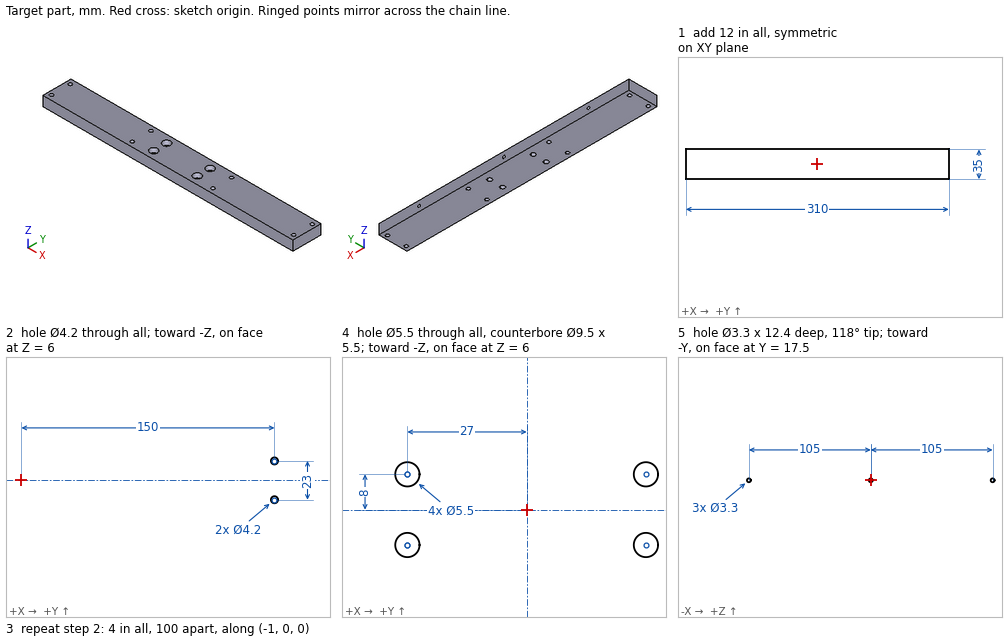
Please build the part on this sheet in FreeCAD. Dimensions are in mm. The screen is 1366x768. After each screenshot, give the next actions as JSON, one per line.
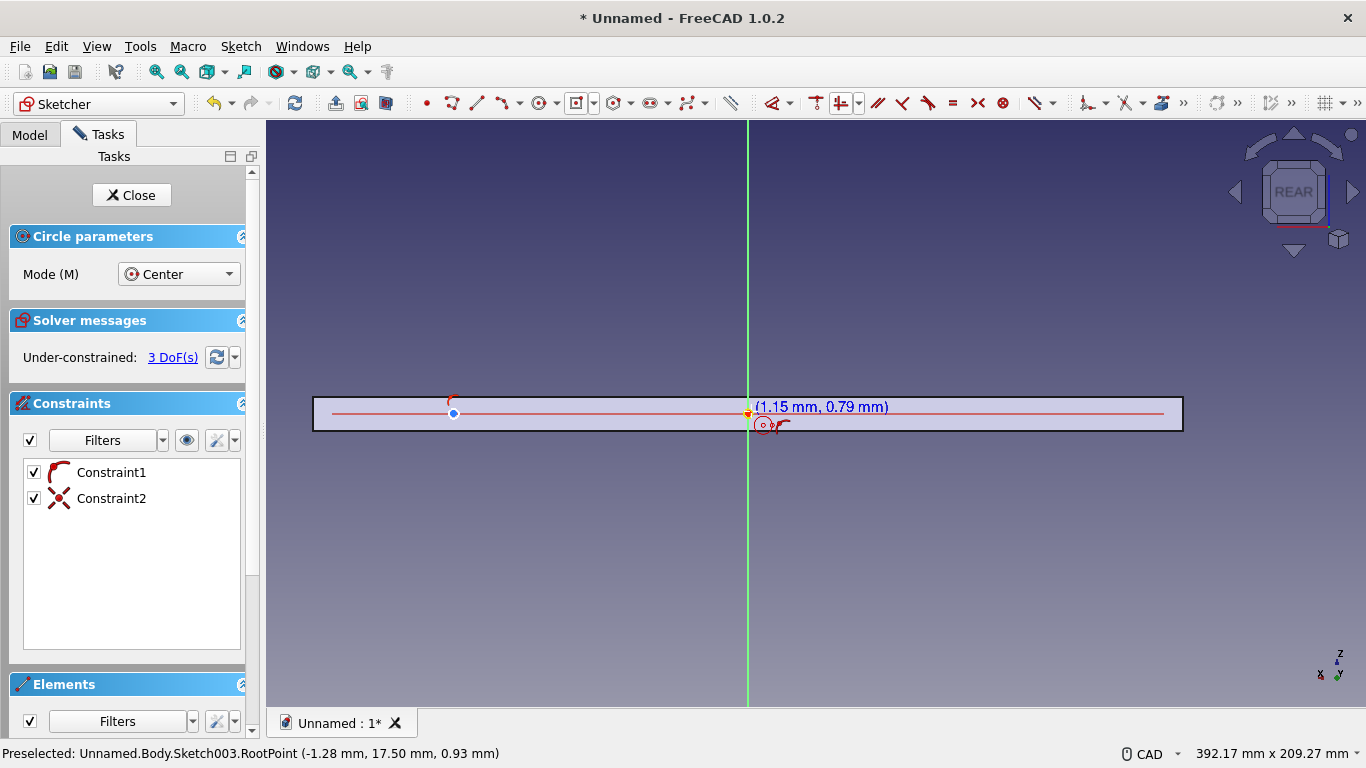
{"action": "scroll", "coordinate": [1043, 414], "scroll_direction": "up", "scroll_amount": 8}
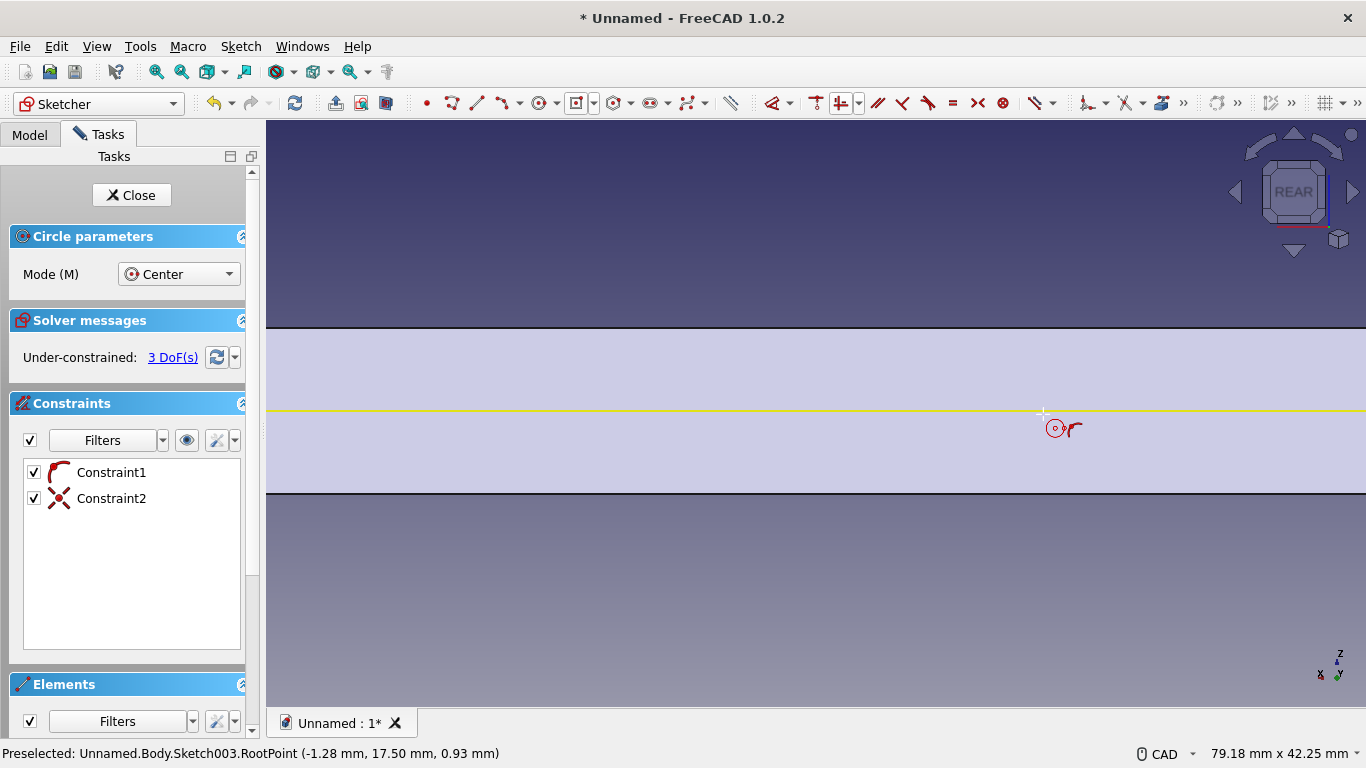
{"action": "scroll", "coordinate": [1043, 414], "scroll_direction": "down", "scroll_amount": 8}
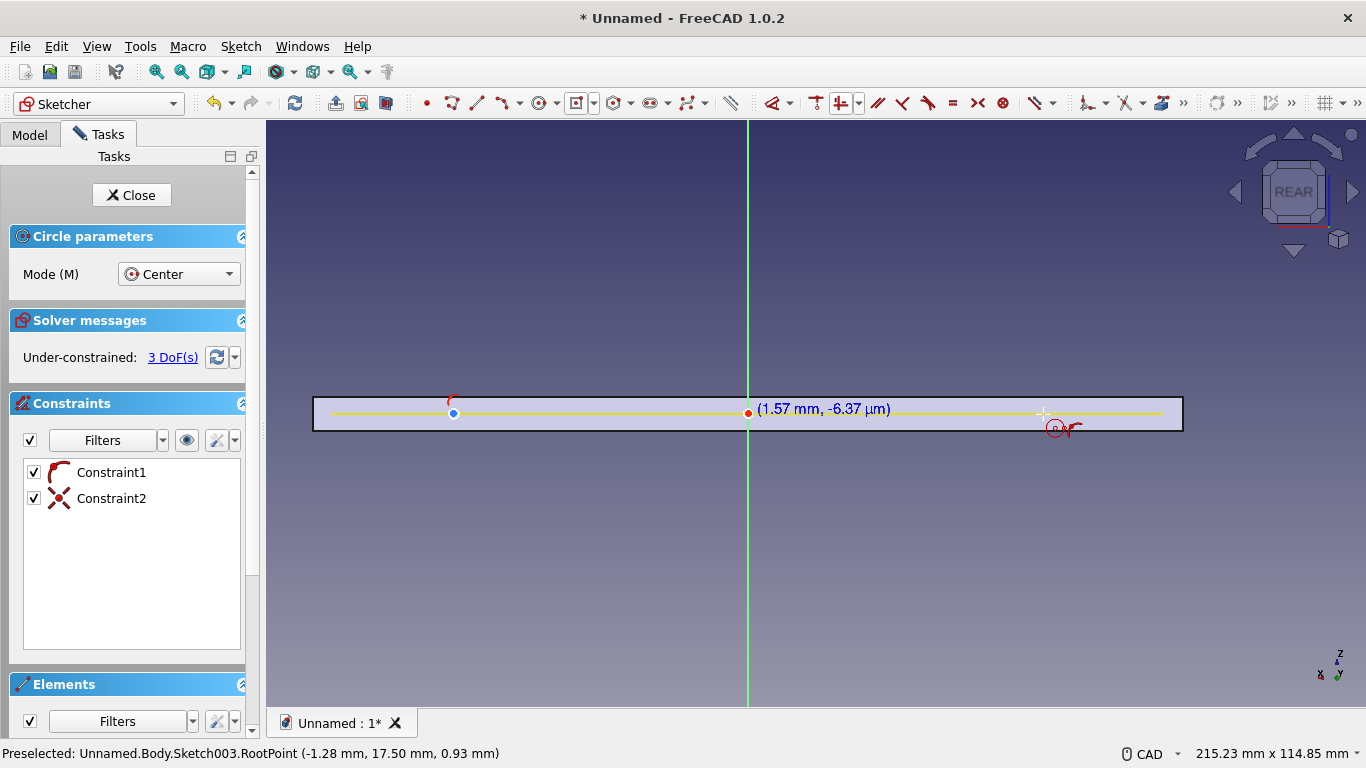
{"action": "left_click", "coordinate": [1043, 414]}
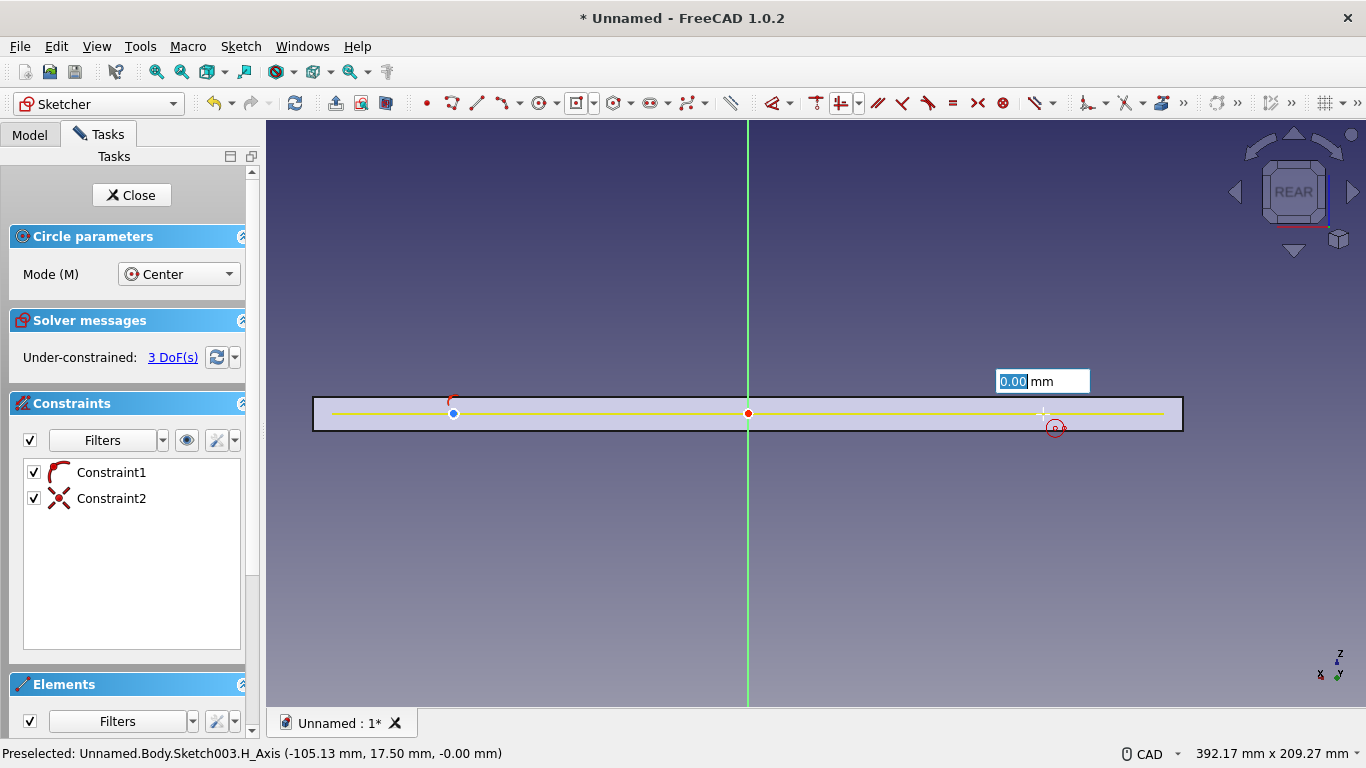
{"action": "scroll", "coordinate": [1041, 418], "scroll_direction": "up", "scroll_amount": 7}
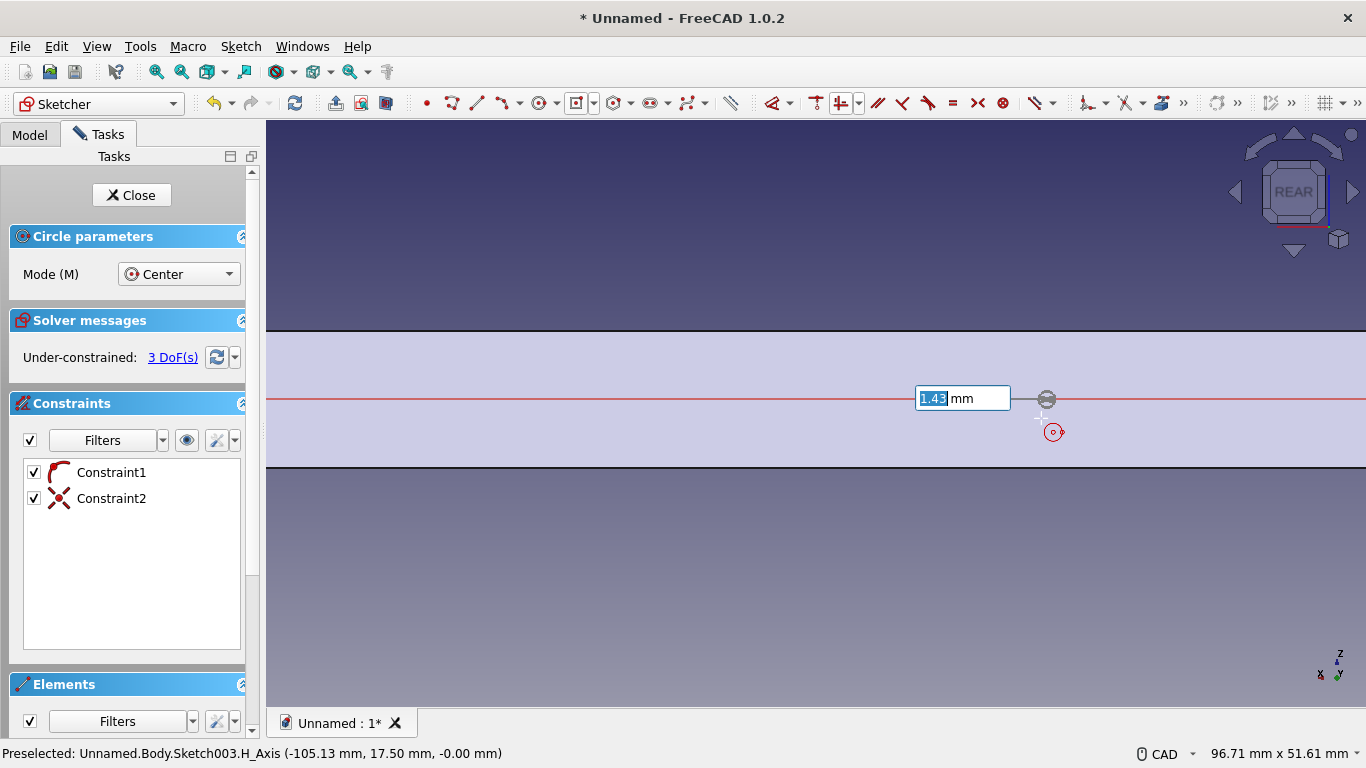
{"action": "left_click", "coordinate": [1039, 417]}
{"action": "key", "text": "Escape"}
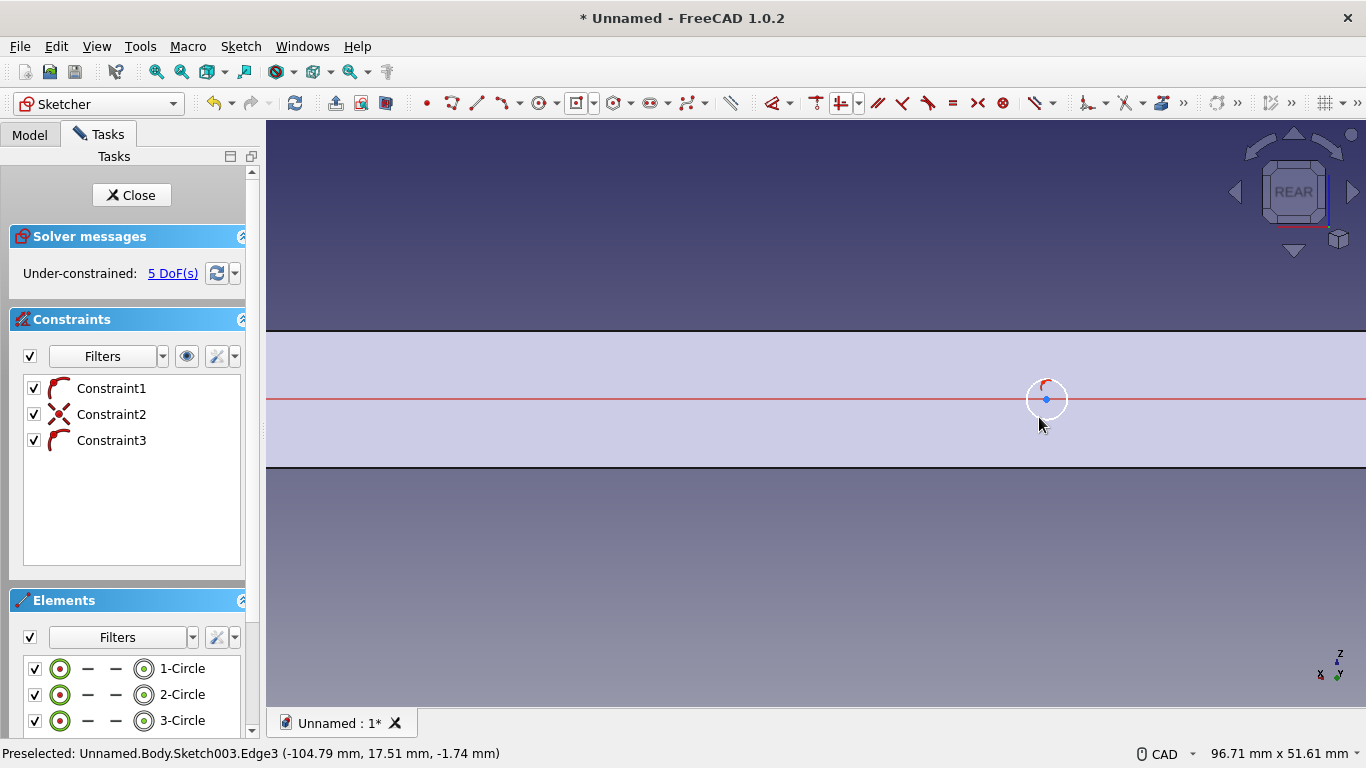
{"action": "scroll", "coordinate": [1041, 418], "scroll_direction": "down", "scroll_amount": 7}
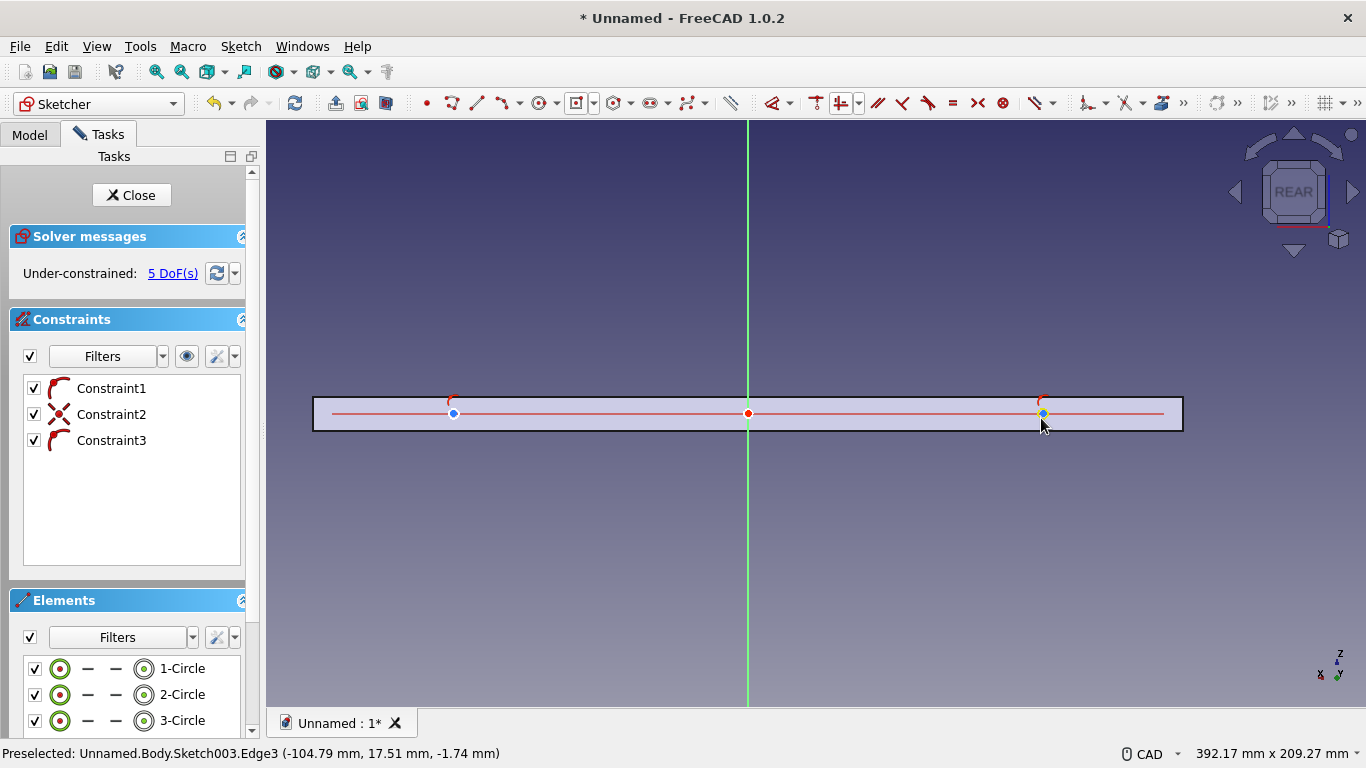
{"action": "scroll", "coordinate": [457, 410], "scroll_direction": "up", "scroll_amount": 7}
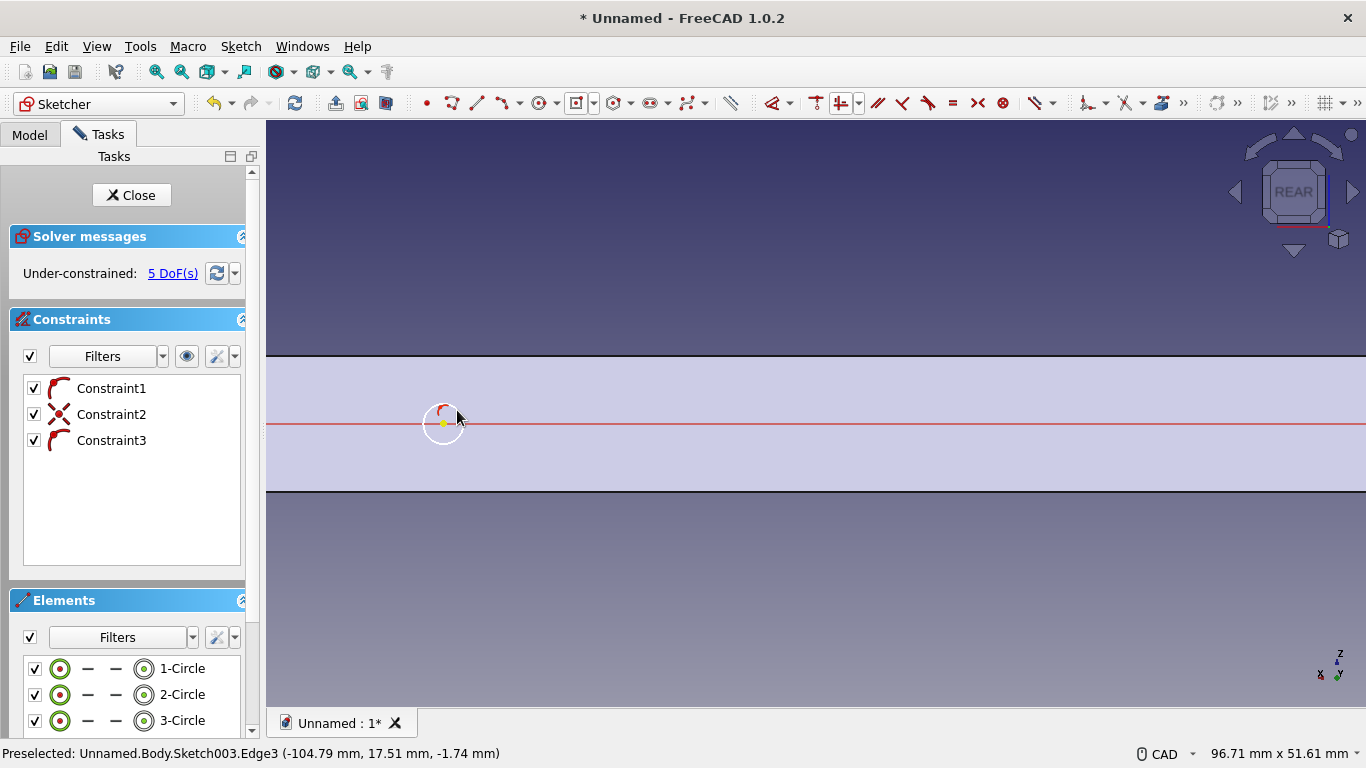
{"action": "left_click", "coordinate": [458, 410]}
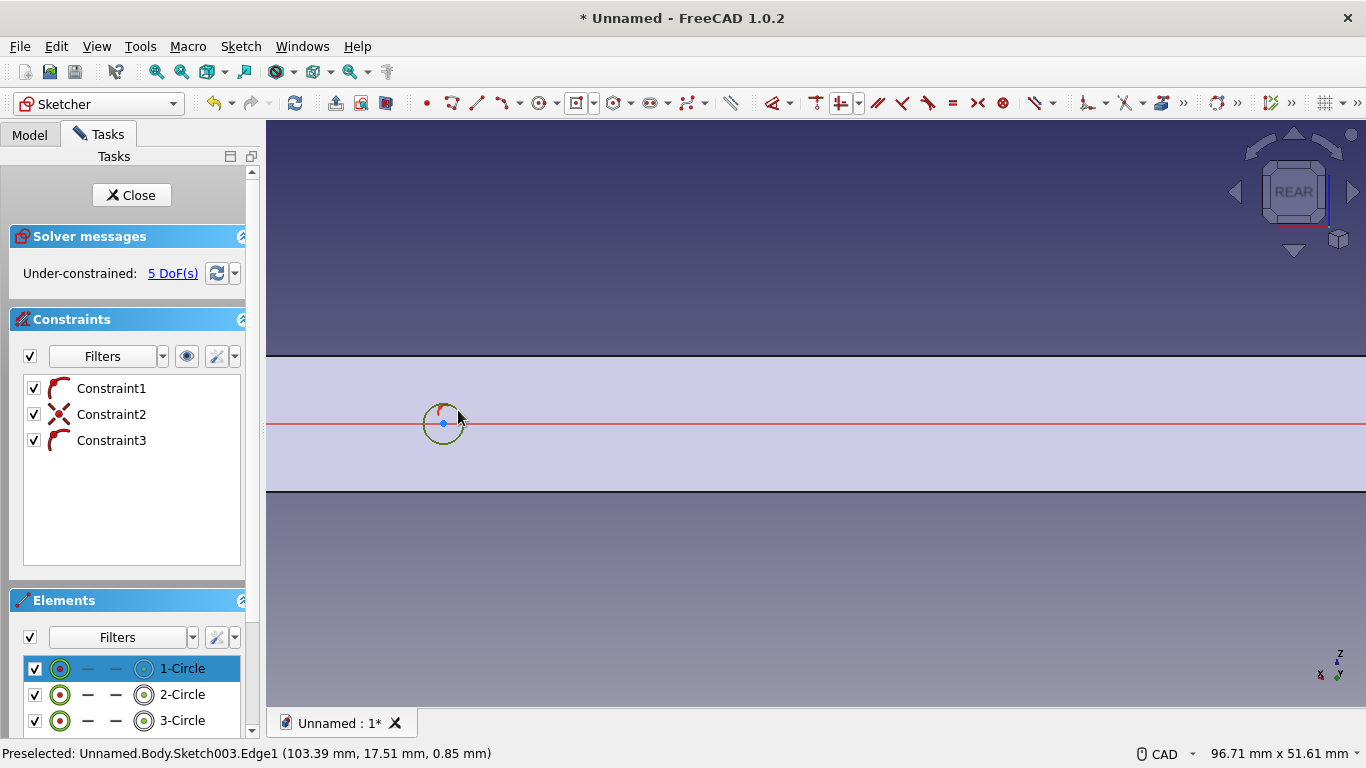
{"action": "scroll", "coordinate": [456, 410], "scroll_direction": "down", "scroll_amount": 7}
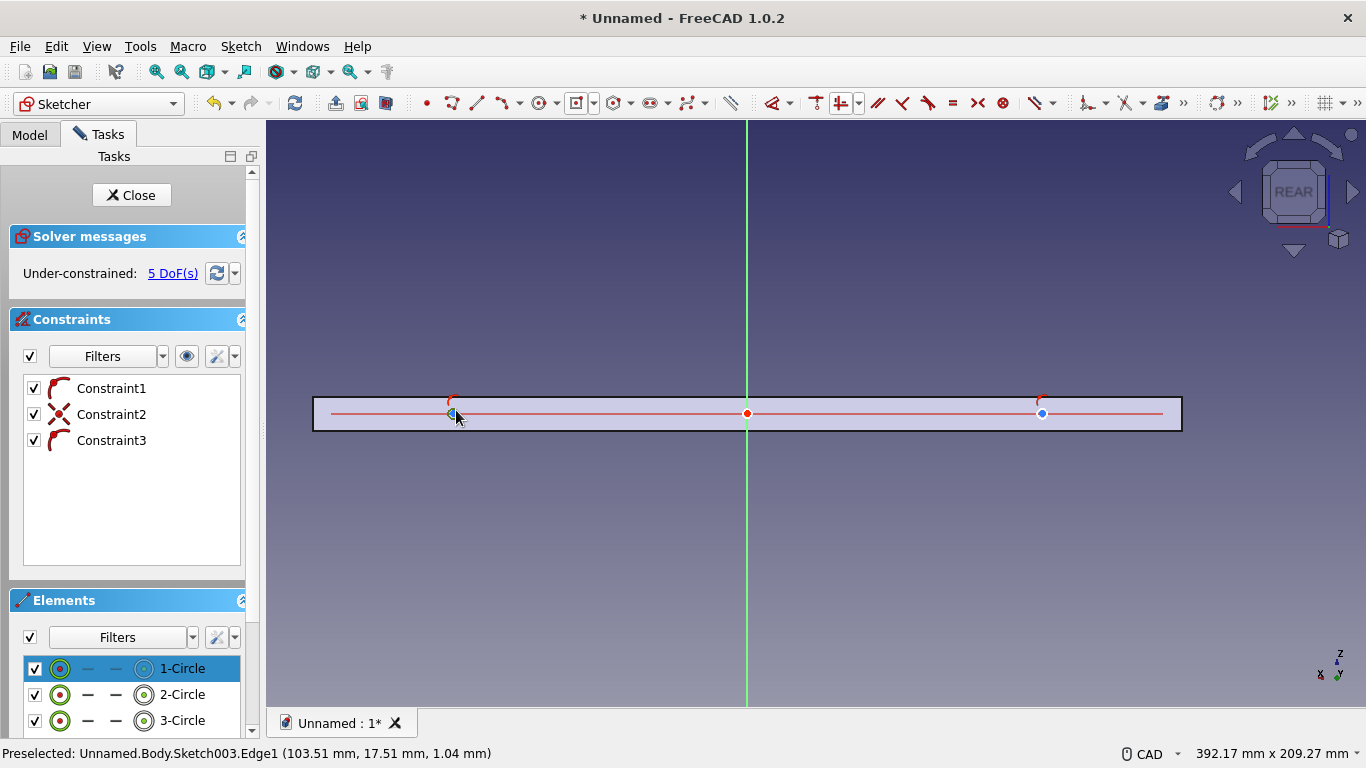
{"action": "scroll", "coordinate": [750, 411], "scroll_direction": "up", "scroll_amount": 8}